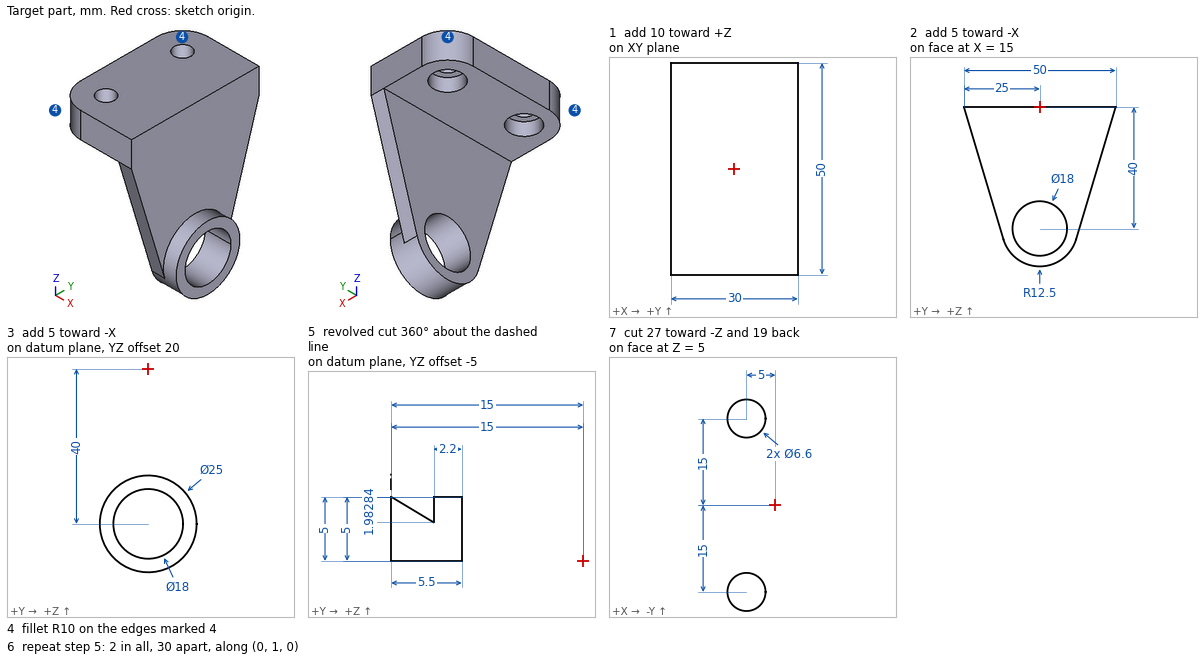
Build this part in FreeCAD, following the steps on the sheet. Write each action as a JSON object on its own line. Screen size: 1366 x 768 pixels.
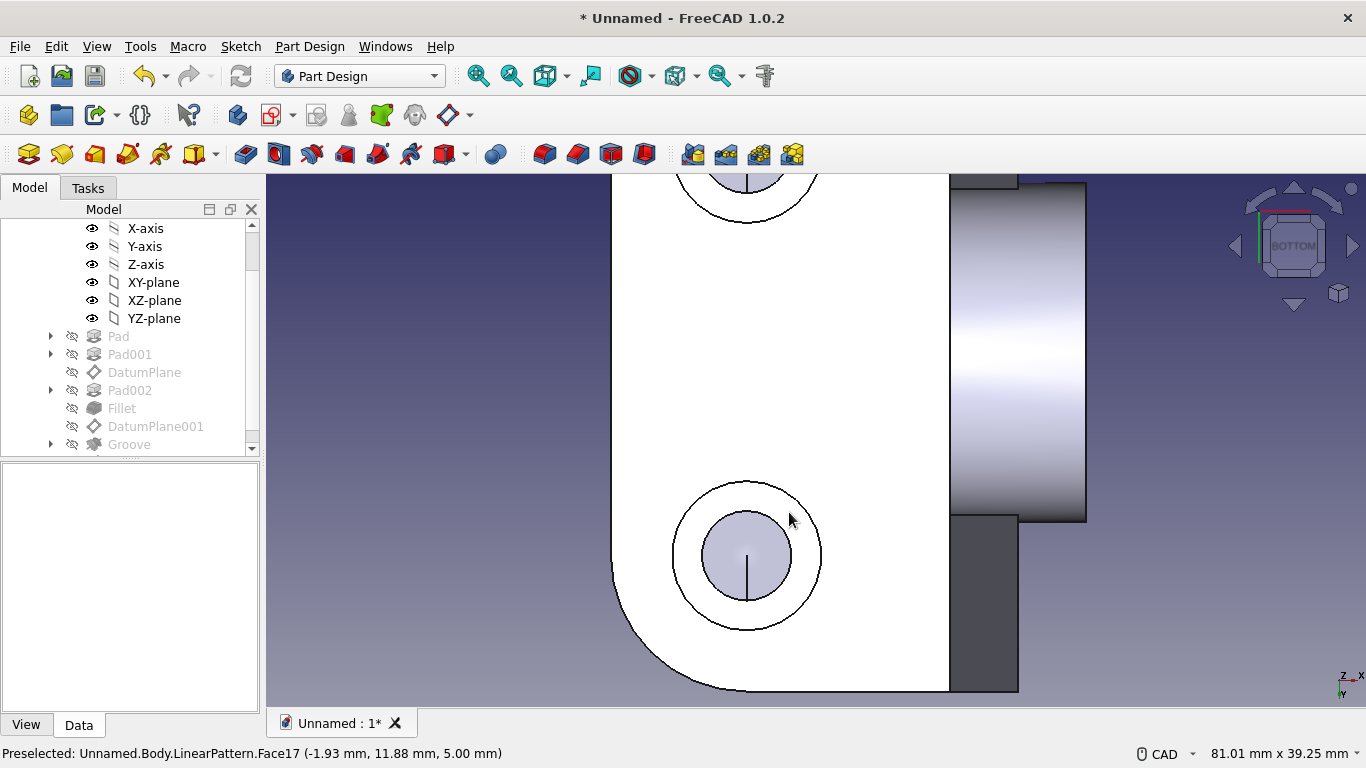
{"action": "left_click", "coordinate": [789, 512]}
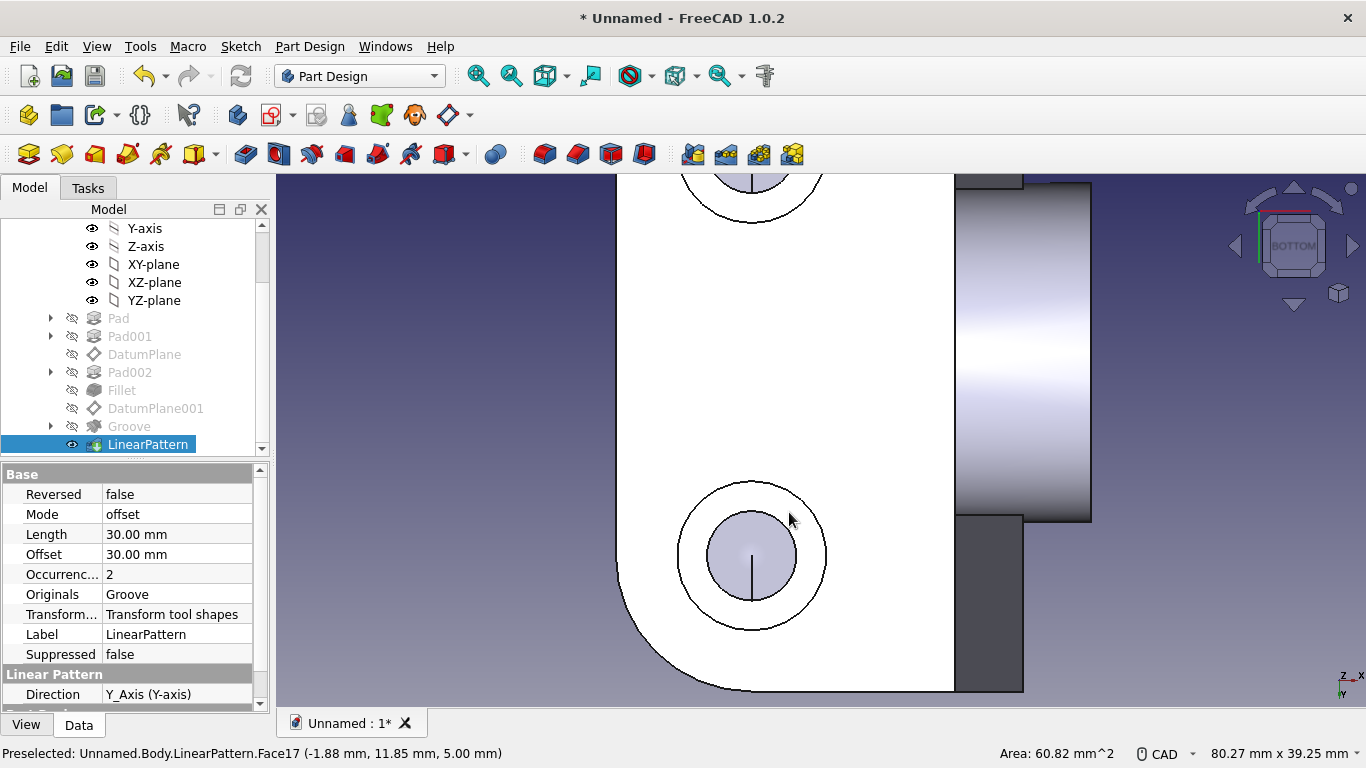
{"action": "left_click", "coordinate": [270, 116]}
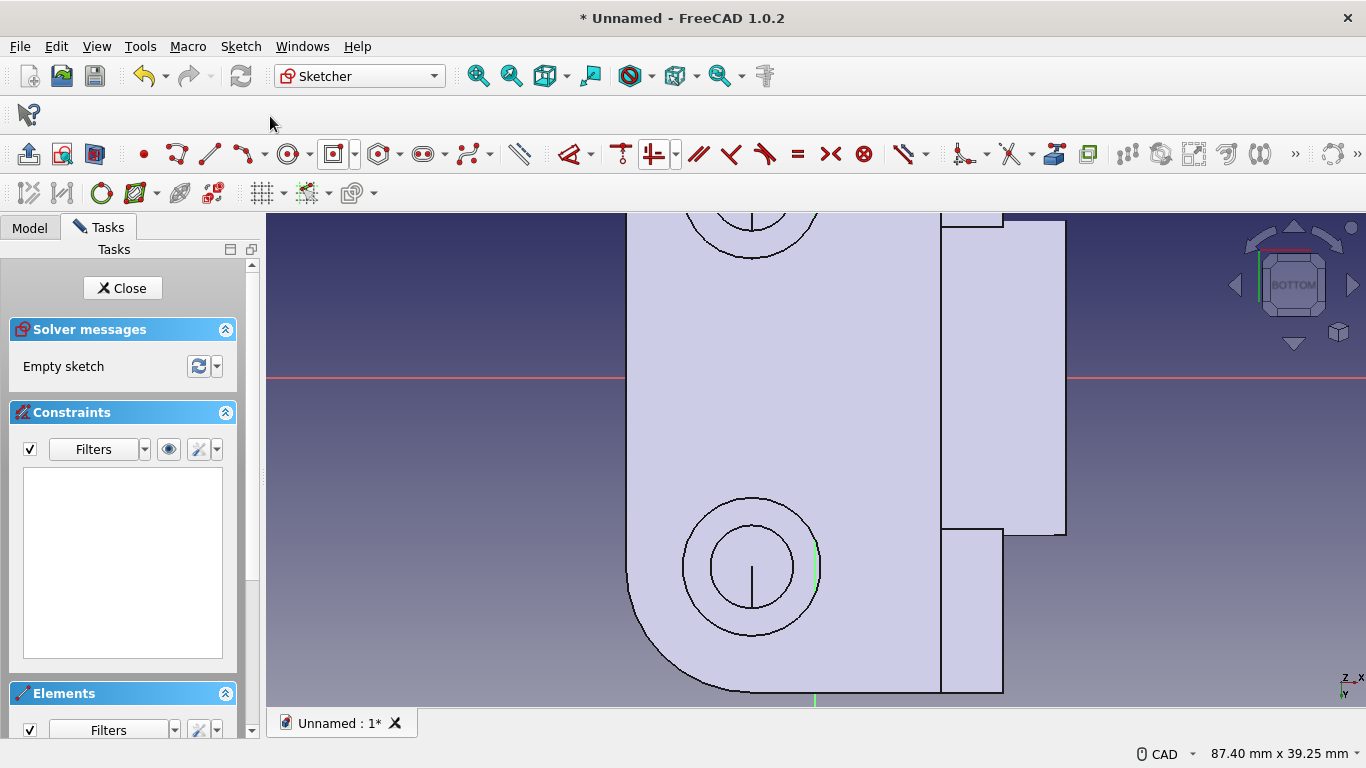
{"action": "scroll", "coordinate": [717, 627], "scroll_direction": "down", "scroll_amount": 2}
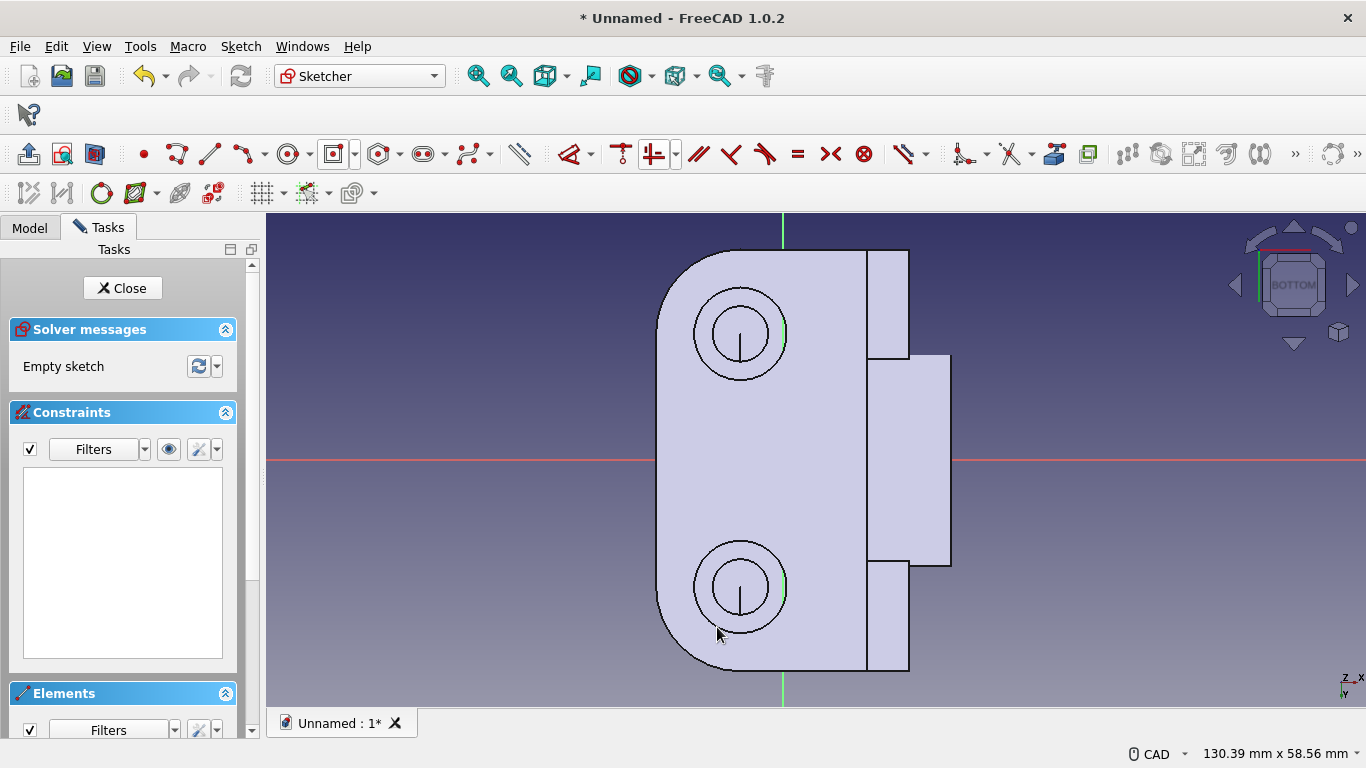
{"action": "left_click", "coordinate": [288, 154]}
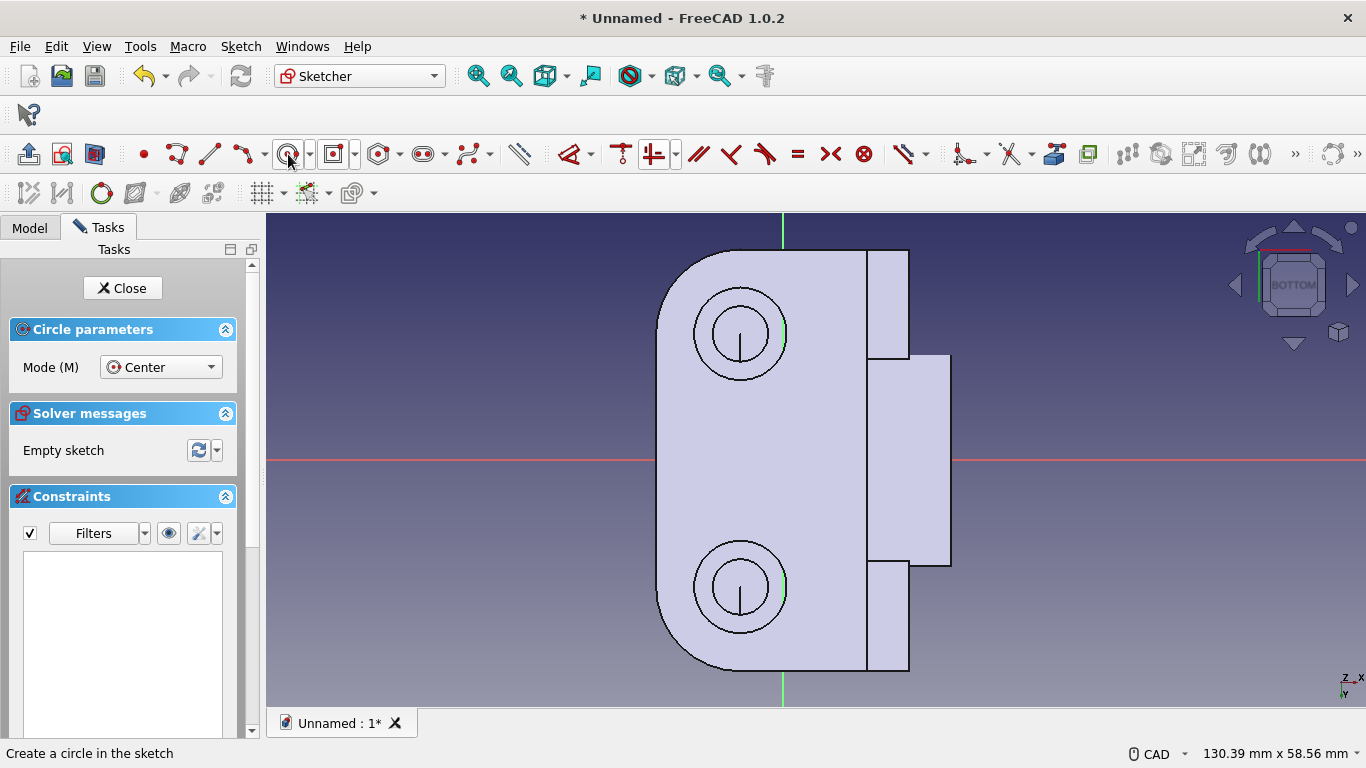
{"action": "left_click", "coordinate": [740, 334]}
{"action": "mouse_move", "coordinate": [760, 314]}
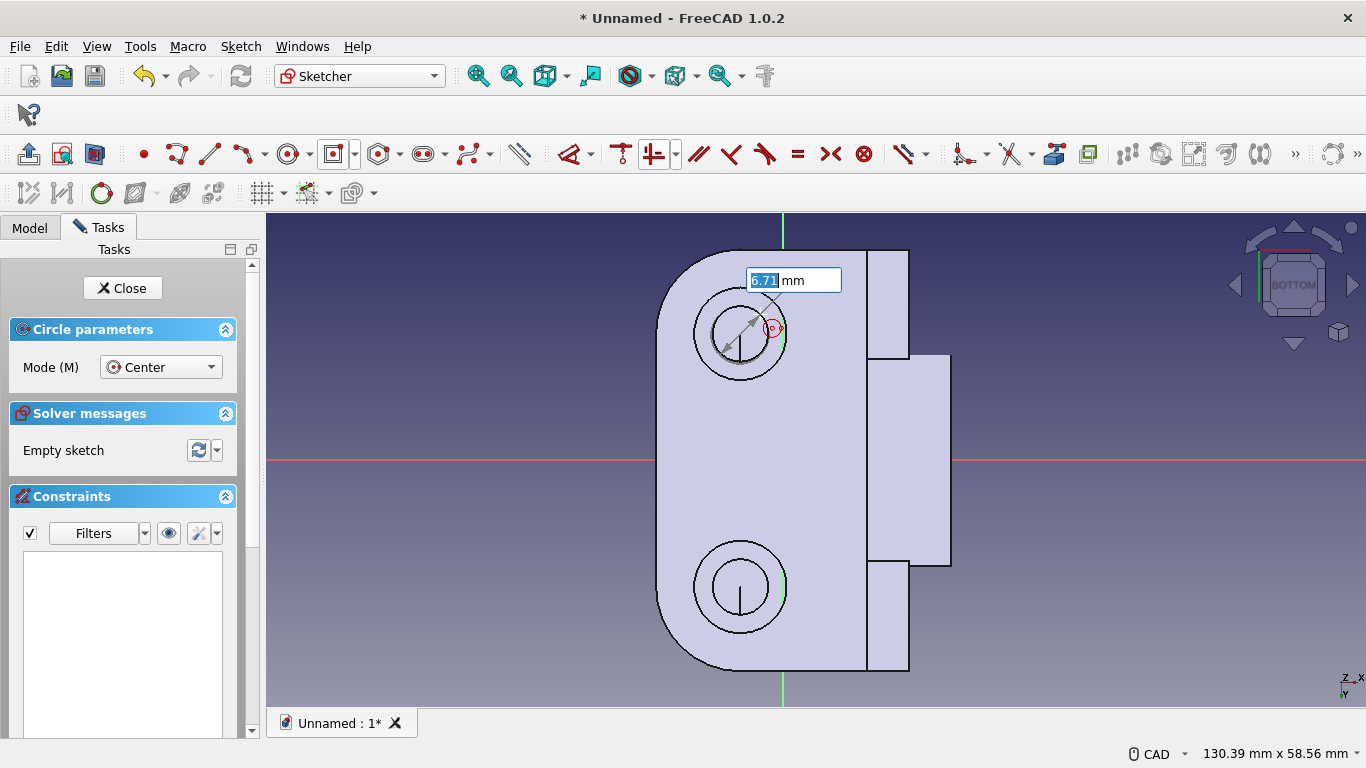
{"action": "type", "text": "6.6"}
{"action": "key", "text": "Return"}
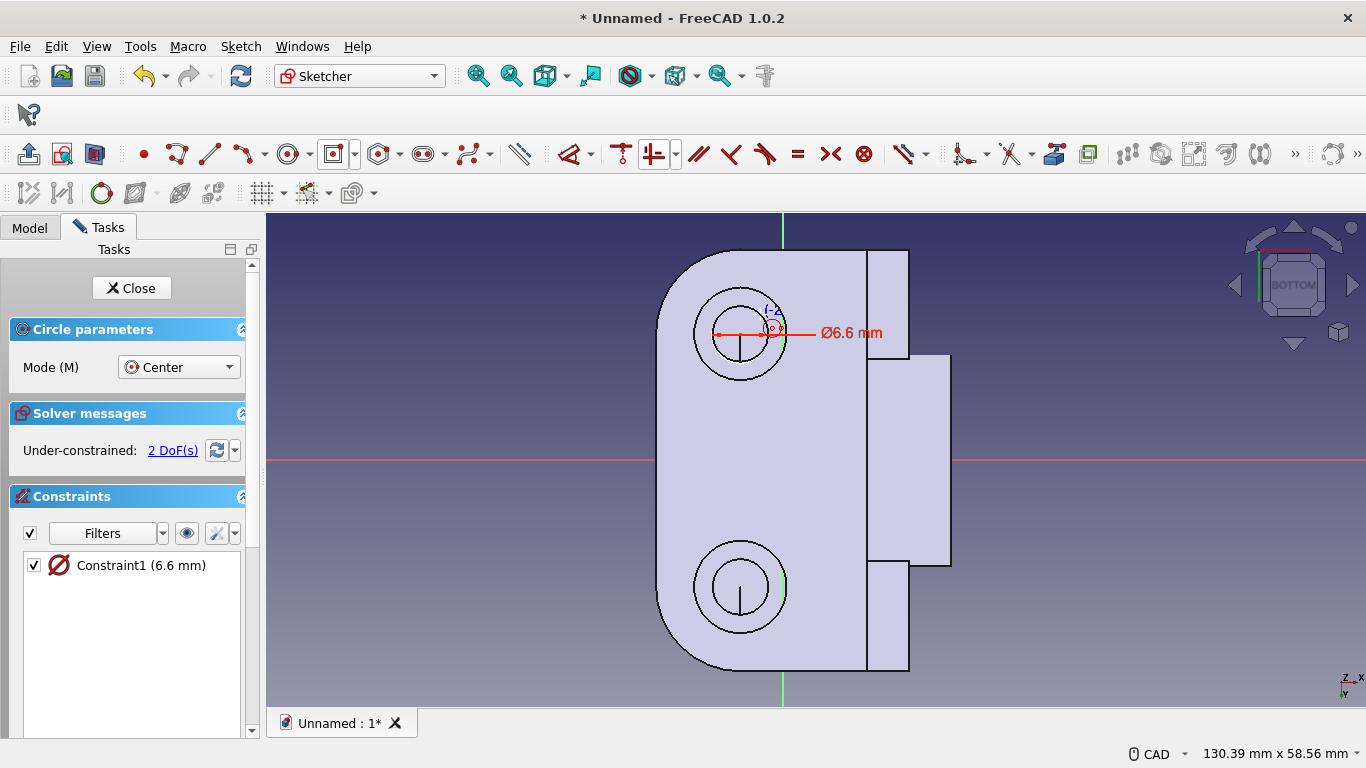
{"action": "left_click", "coordinate": [740, 587]}
{"action": "mouse_move", "coordinate": [760, 567]}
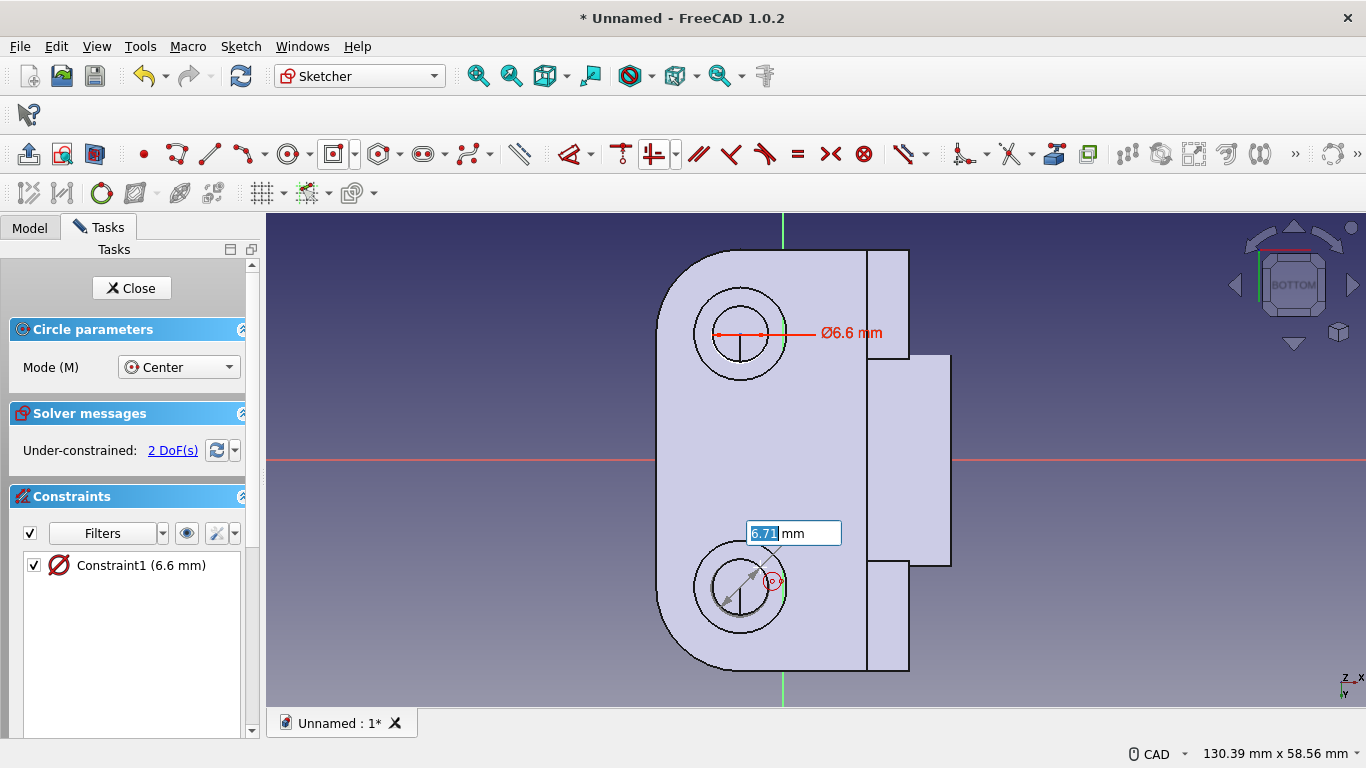
{"action": "type", "text": "6.6"}
{"action": "key", "text": "Return"}
{"action": "key", "text": "Escape"}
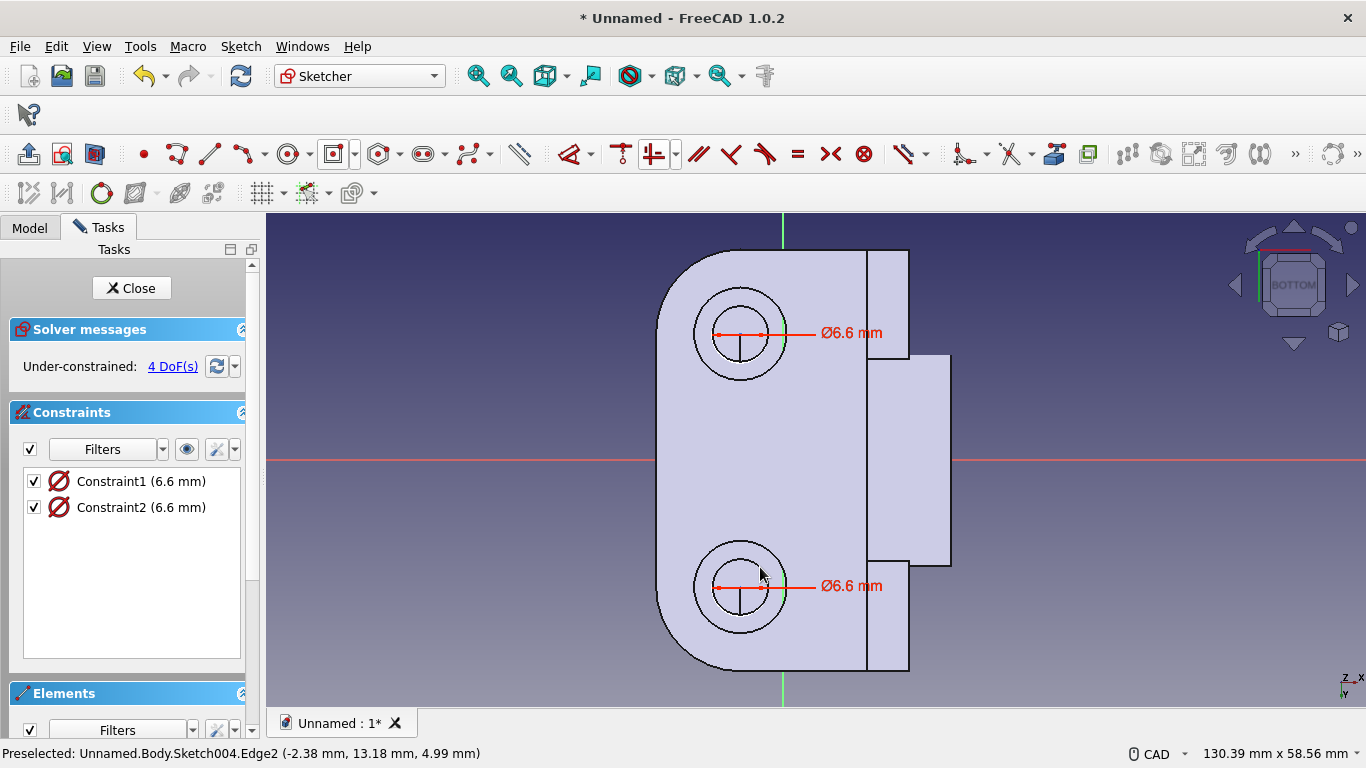
{"action": "left_click", "coordinate": [740, 335]}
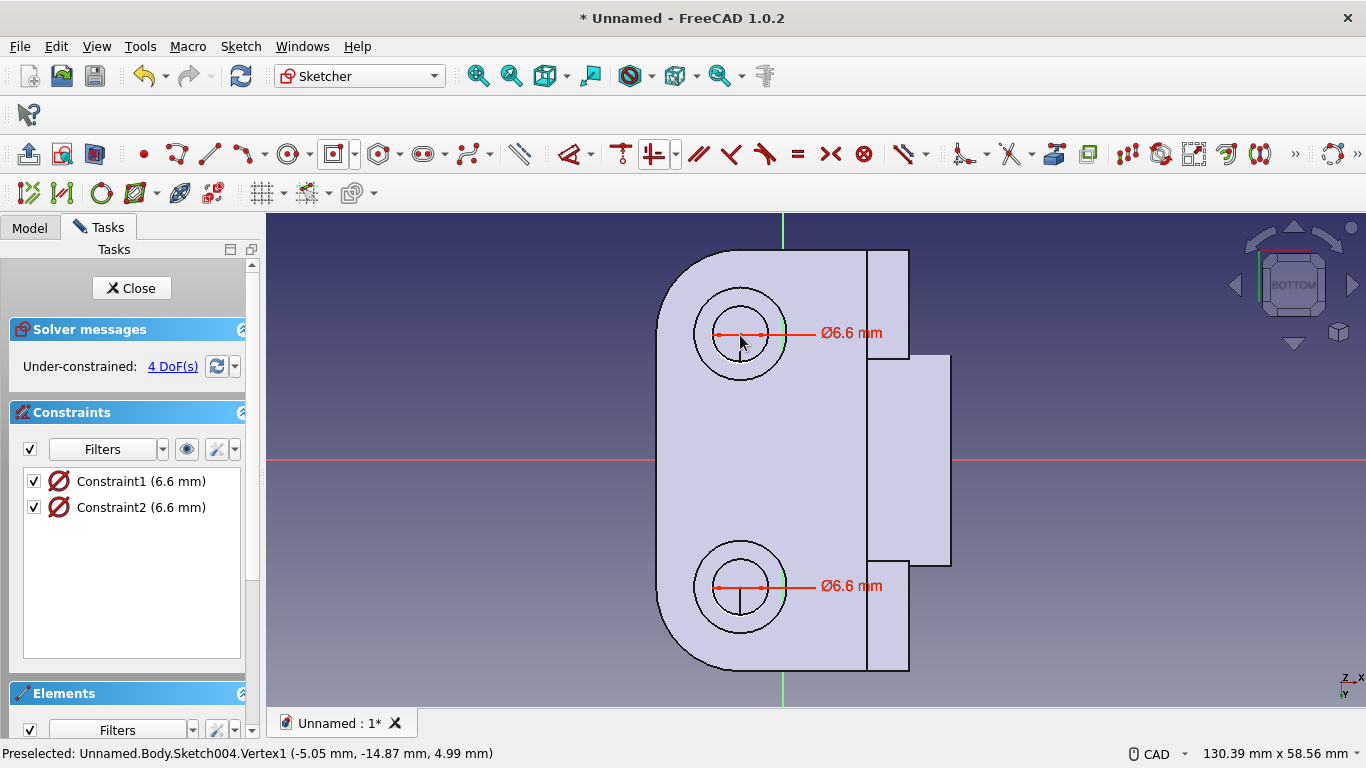
{"action": "left_click", "coordinate": [740, 588]}